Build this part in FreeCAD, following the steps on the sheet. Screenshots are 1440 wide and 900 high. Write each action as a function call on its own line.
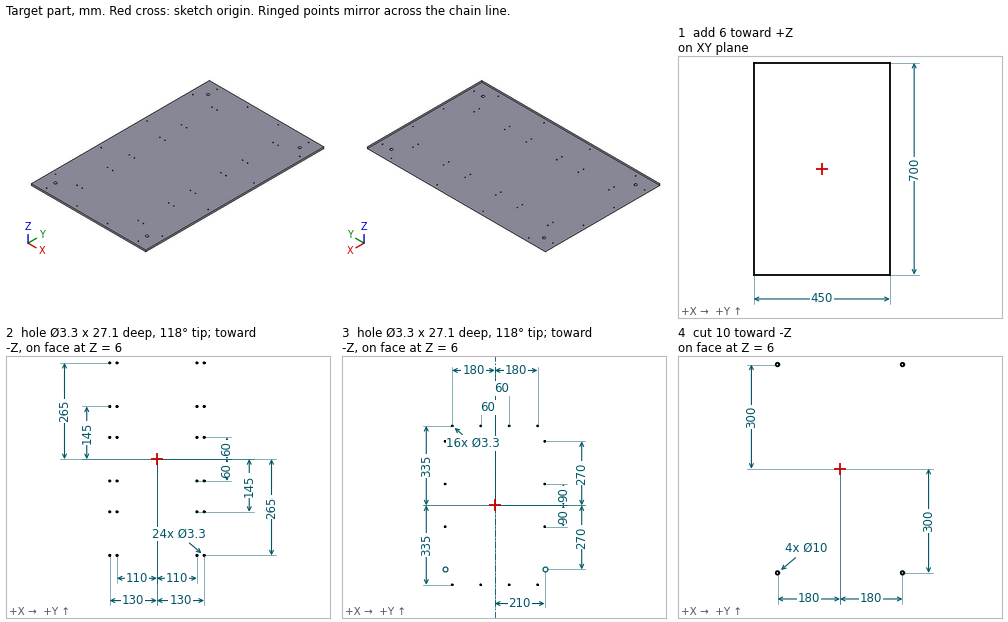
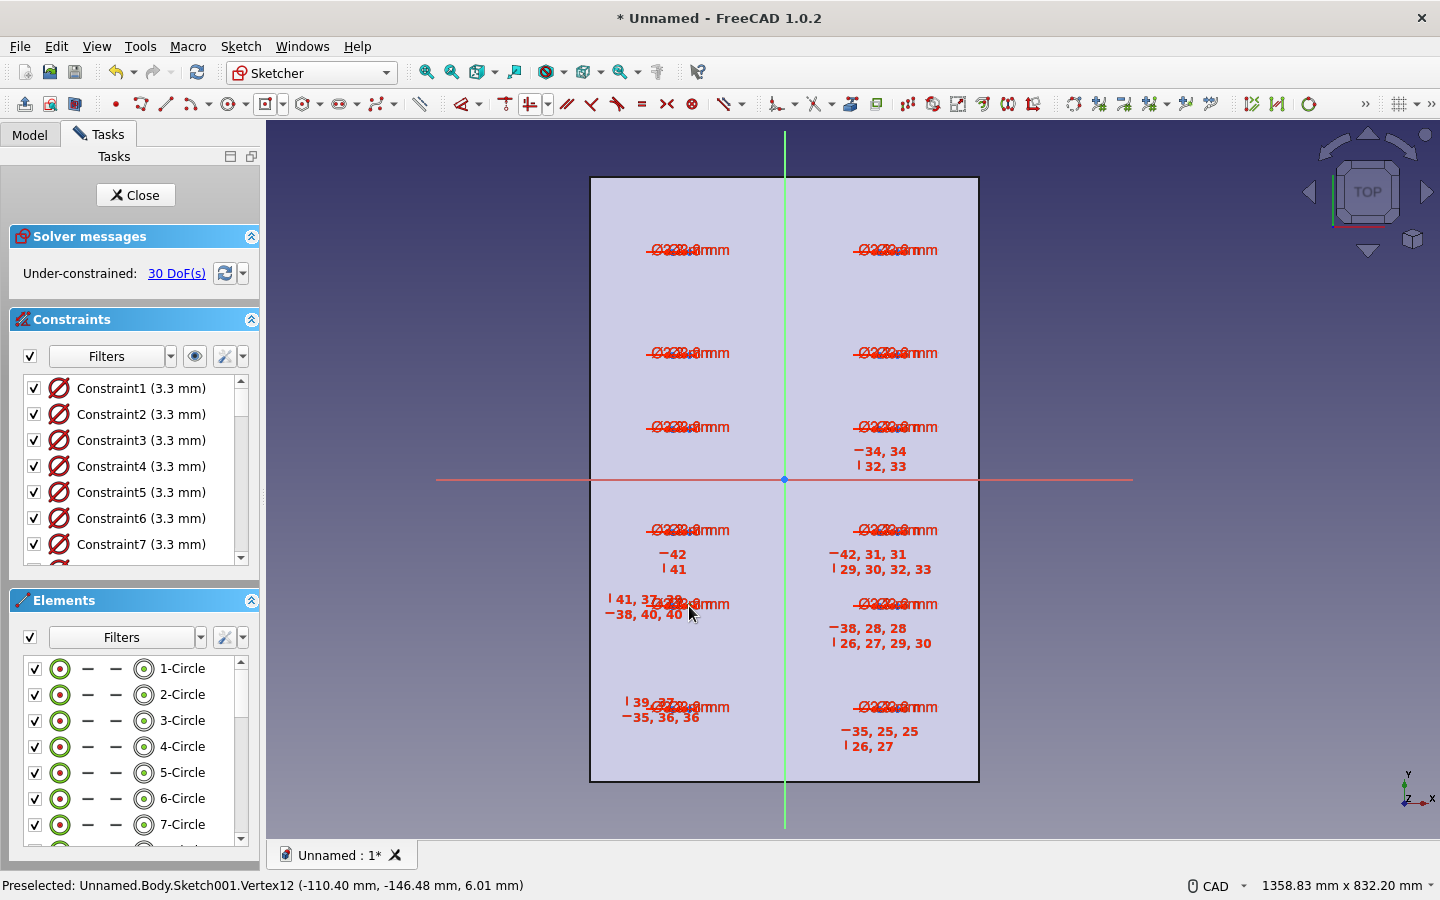
click(689, 532)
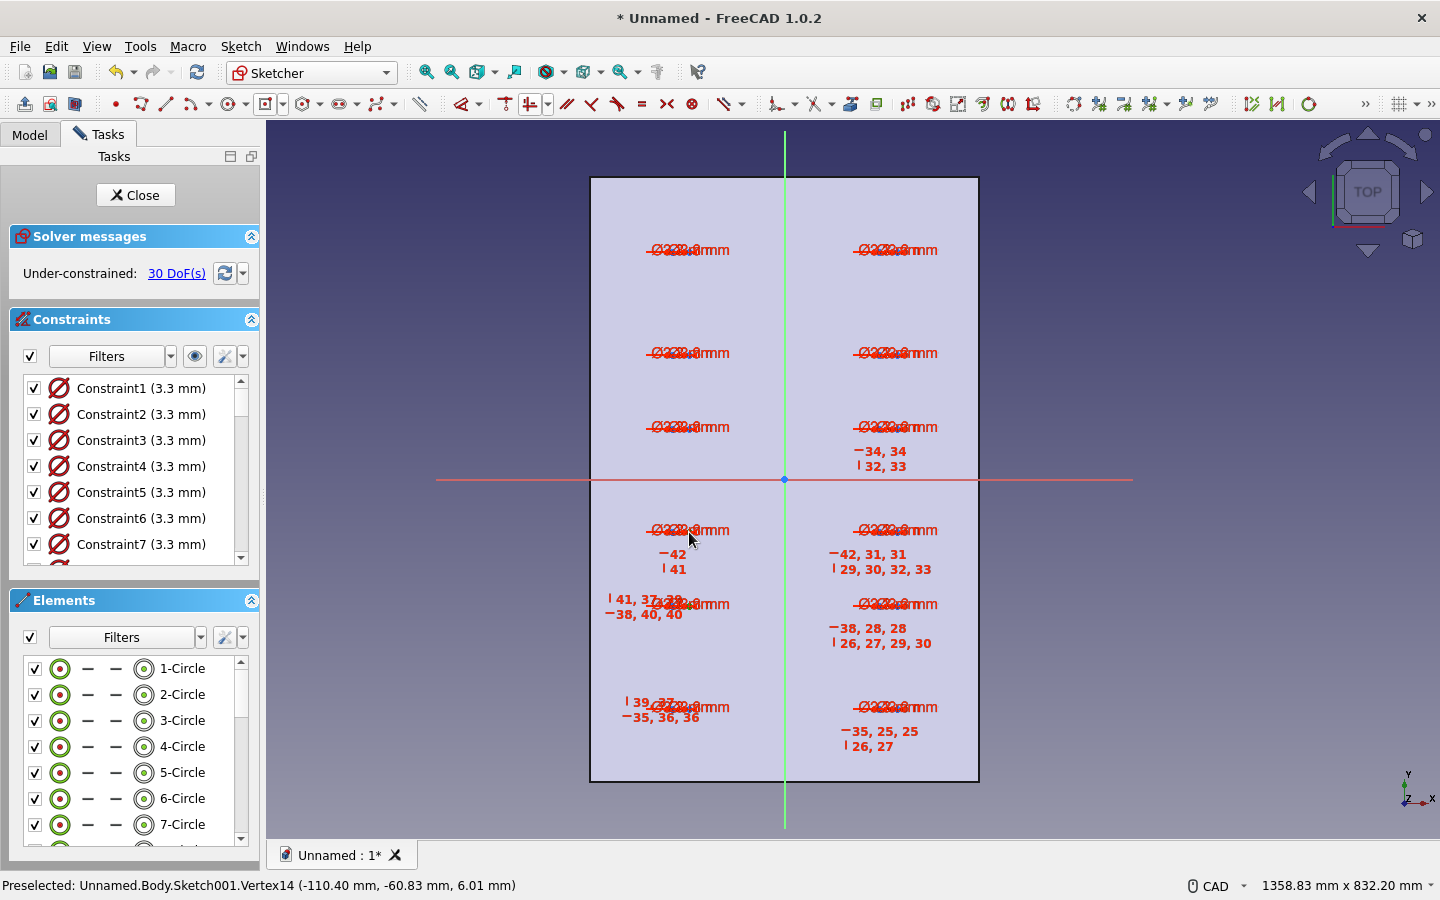
click(548, 104)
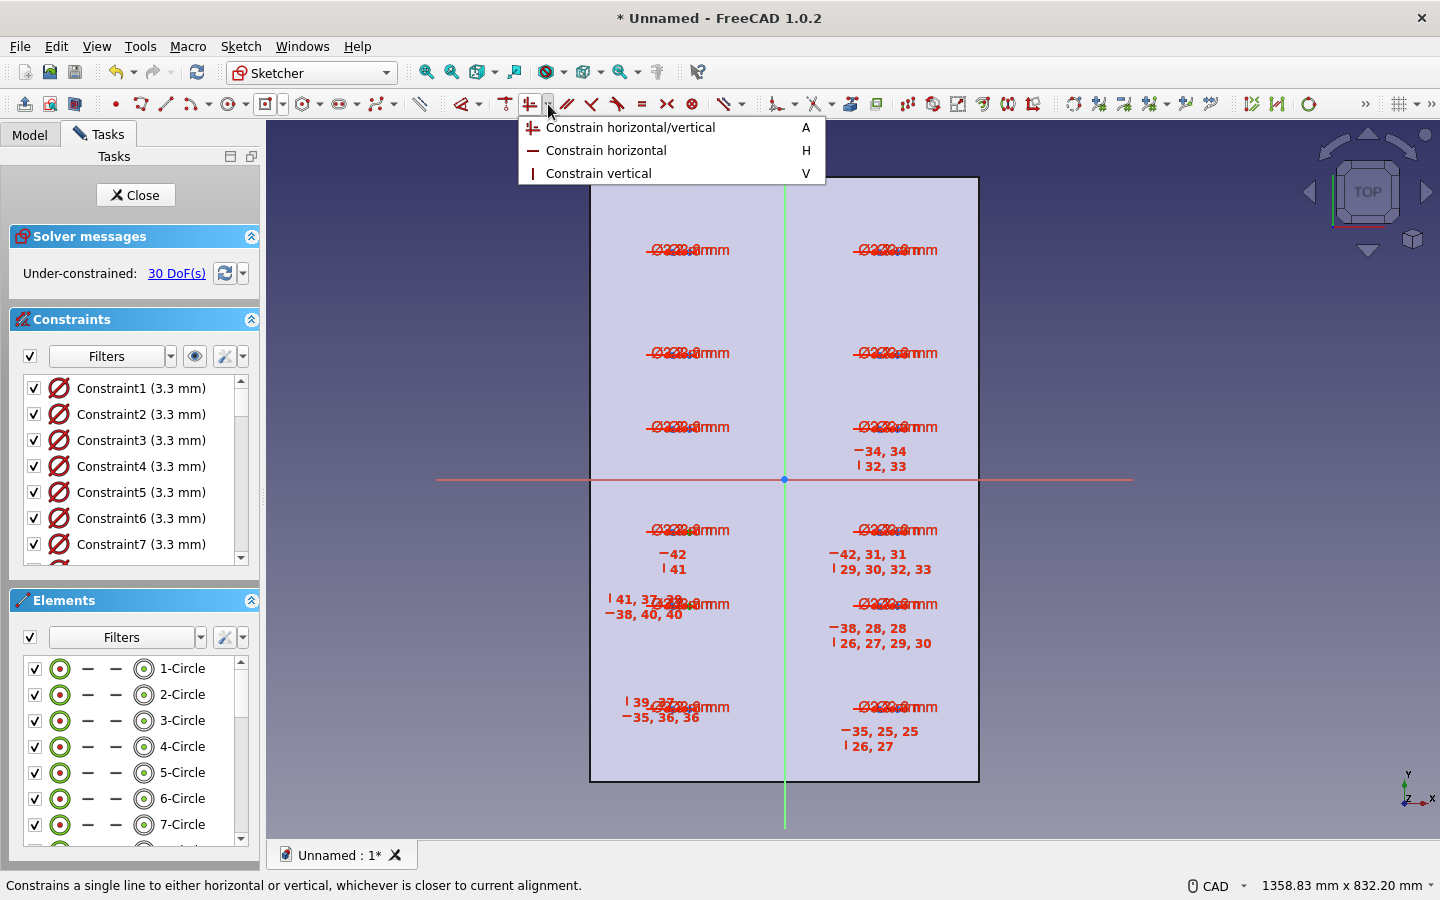
click(672, 174)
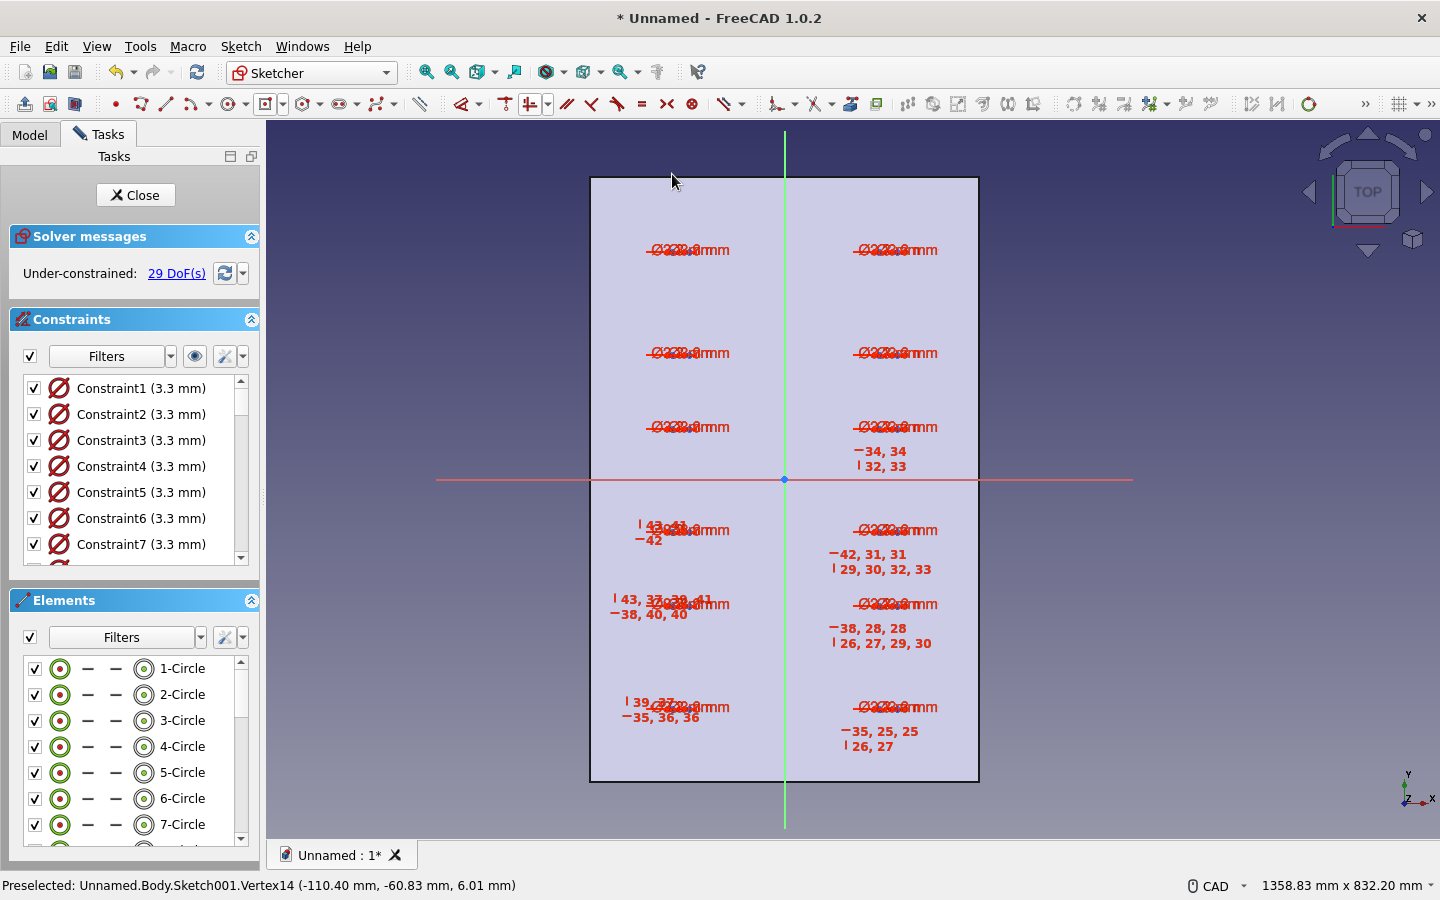
scroll(672, 532, up, 4)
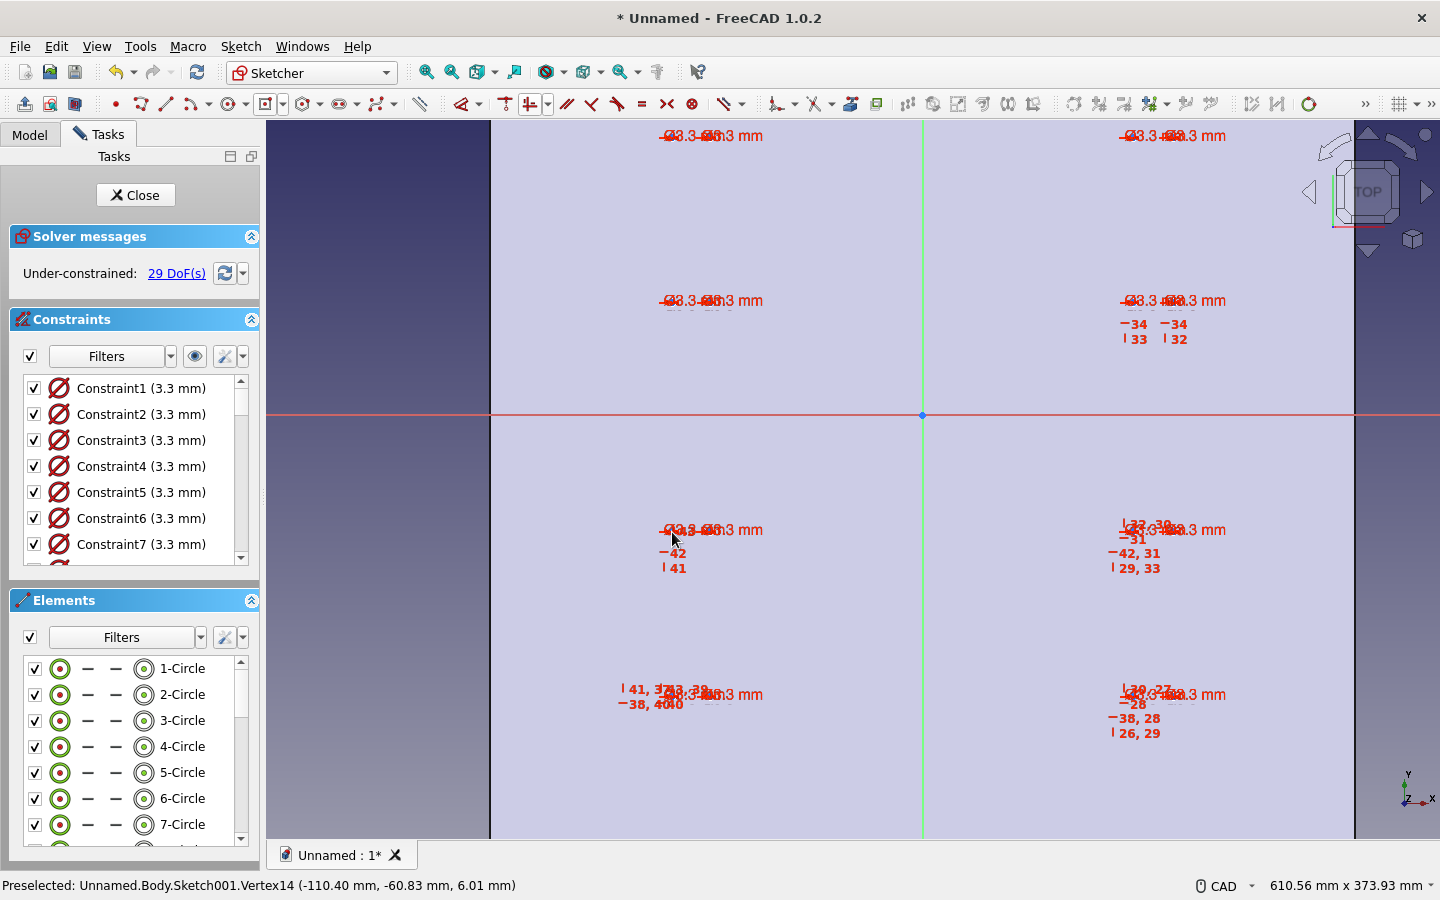
scroll(672, 532, up, 4)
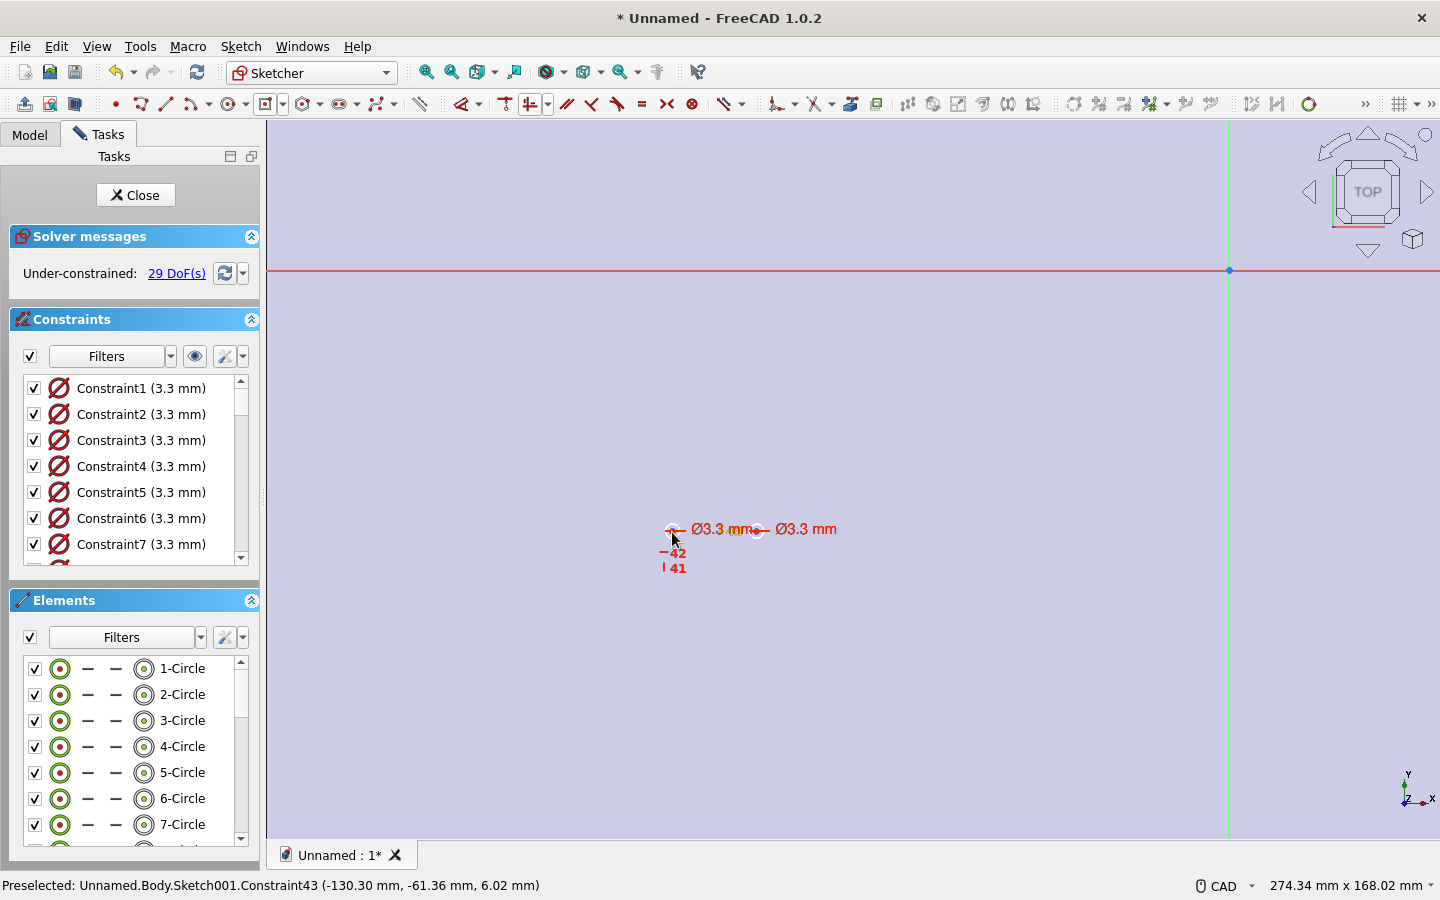
click(673, 531)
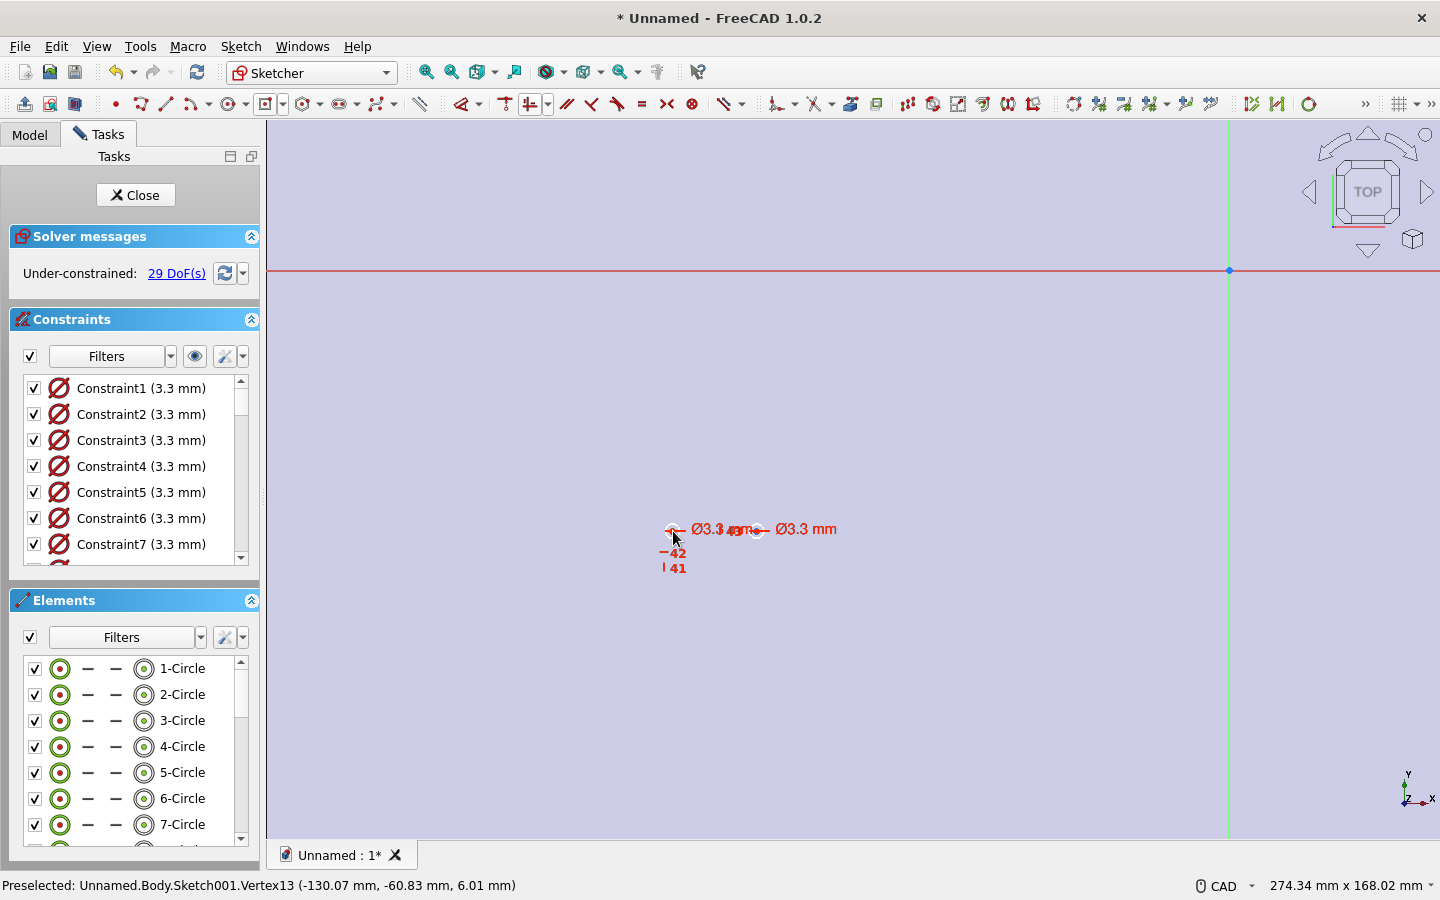
scroll(672, 532, down, 8)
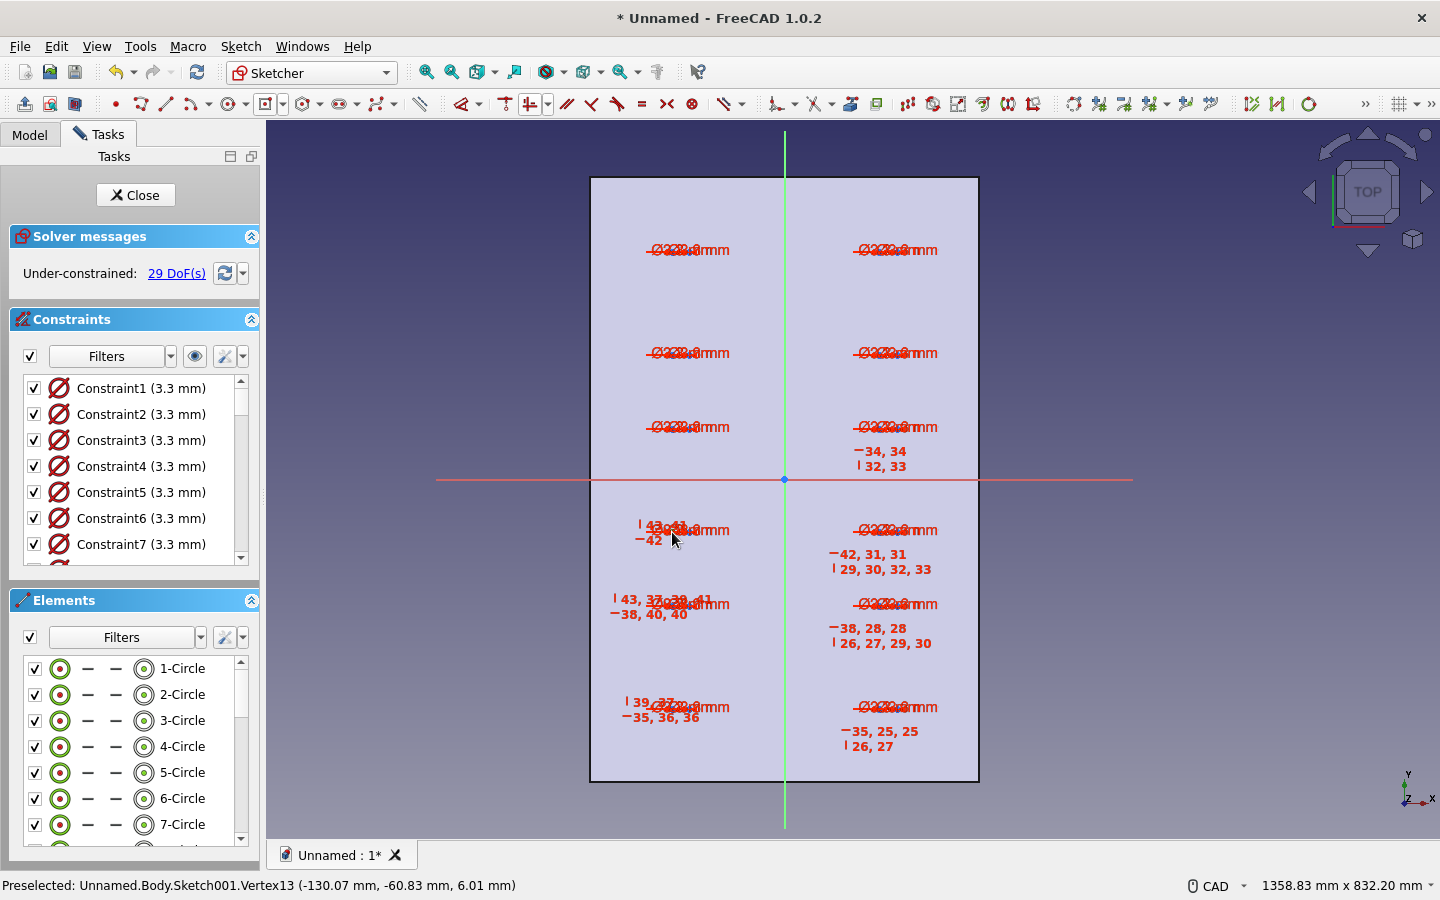
click(689, 532)